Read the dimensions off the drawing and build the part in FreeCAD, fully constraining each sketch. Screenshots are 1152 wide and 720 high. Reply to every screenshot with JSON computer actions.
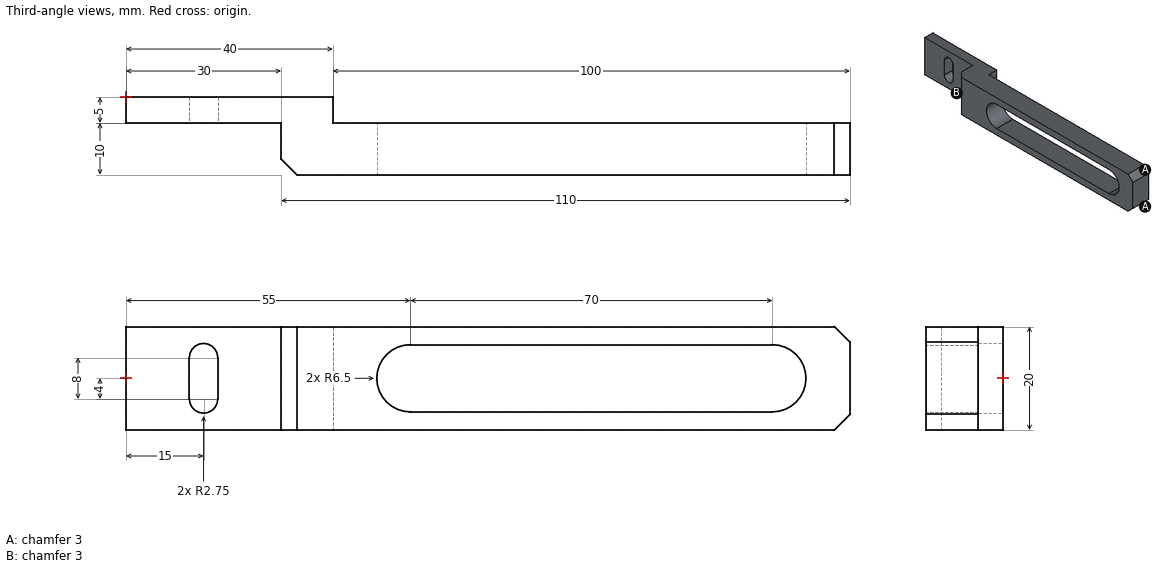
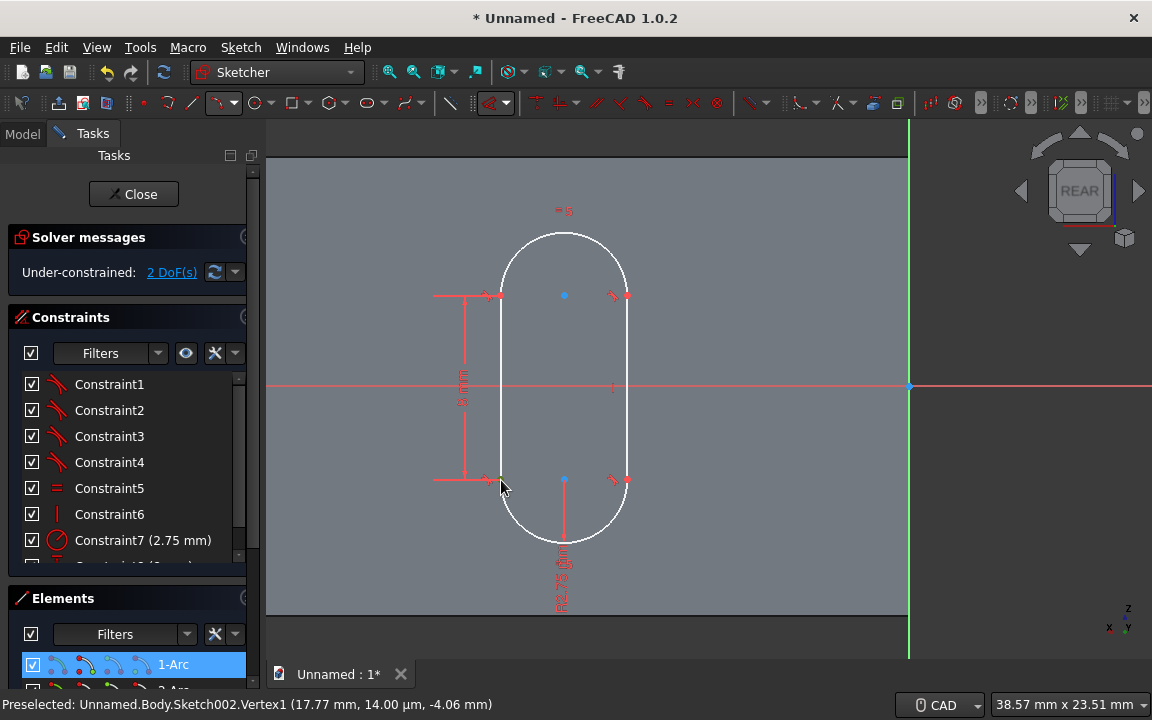
{"action": "key", "text": "i"}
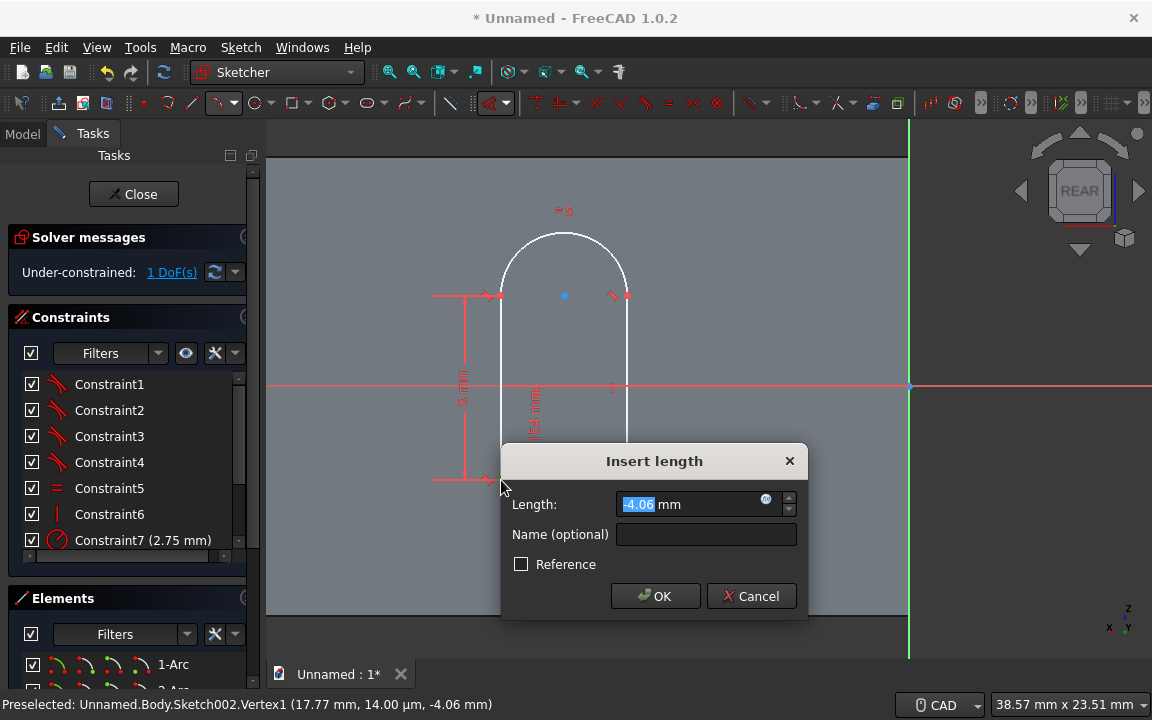
{"action": "type", "text": "-4"}
{"action": "key", "text": "Return"}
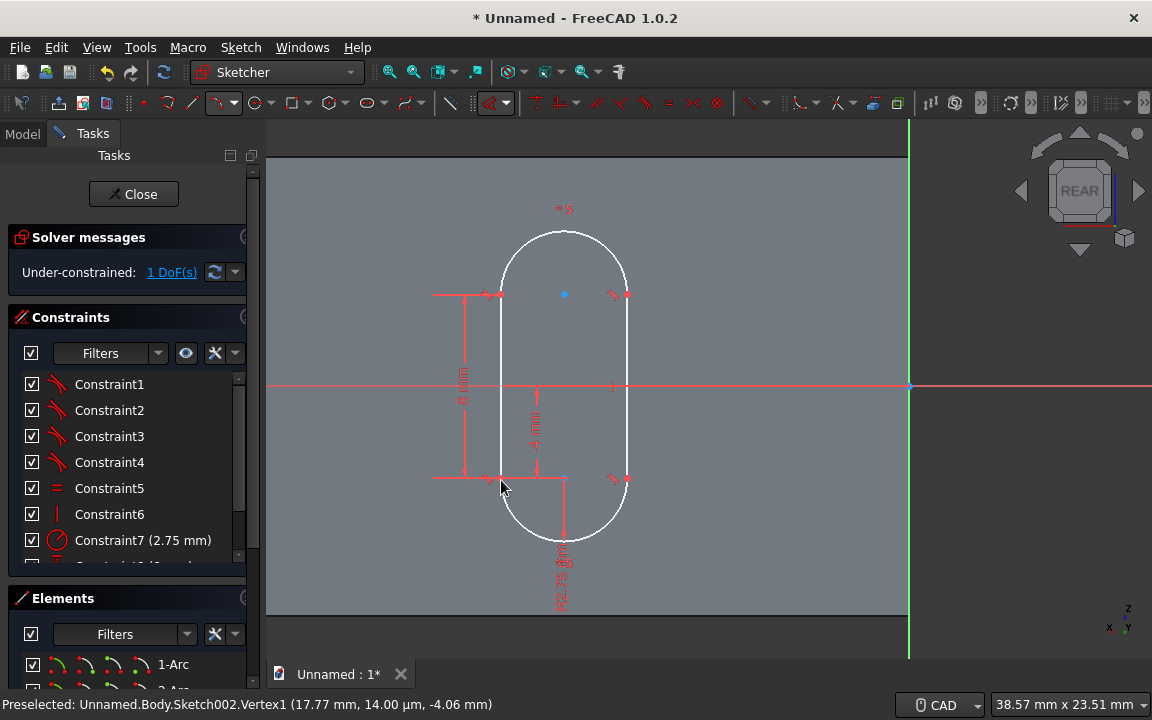
{"action": "left_click", "coordinate": [564, 478]}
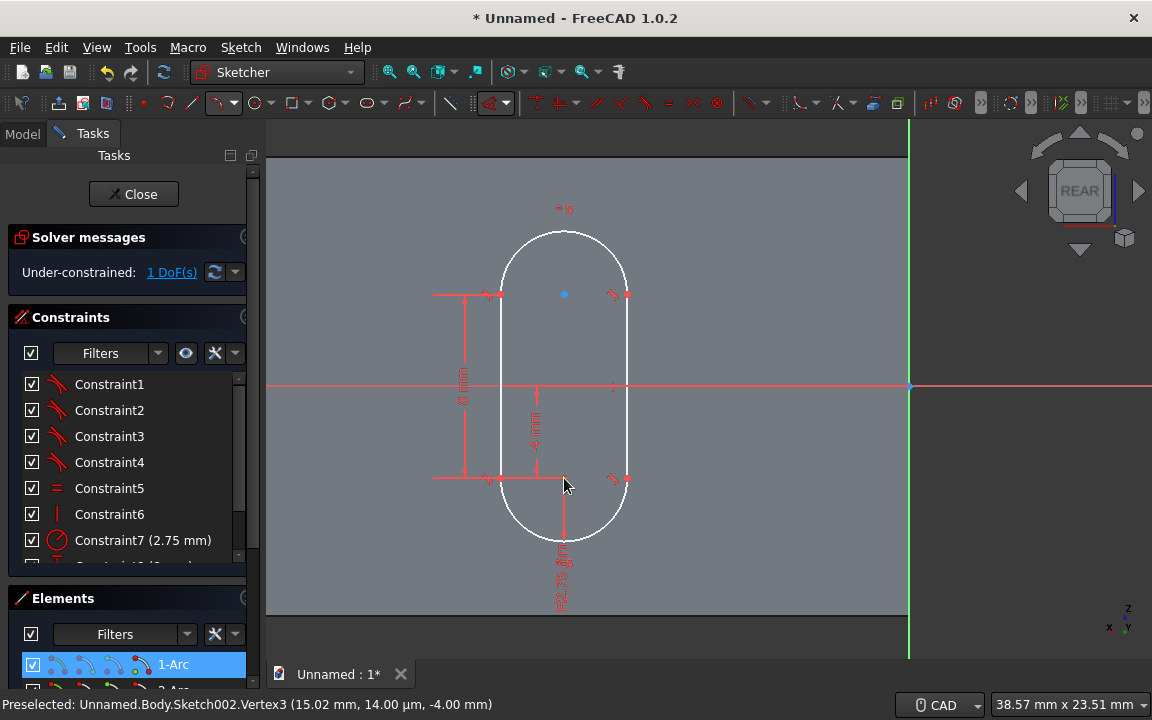
{"action": "key", "text": "l"}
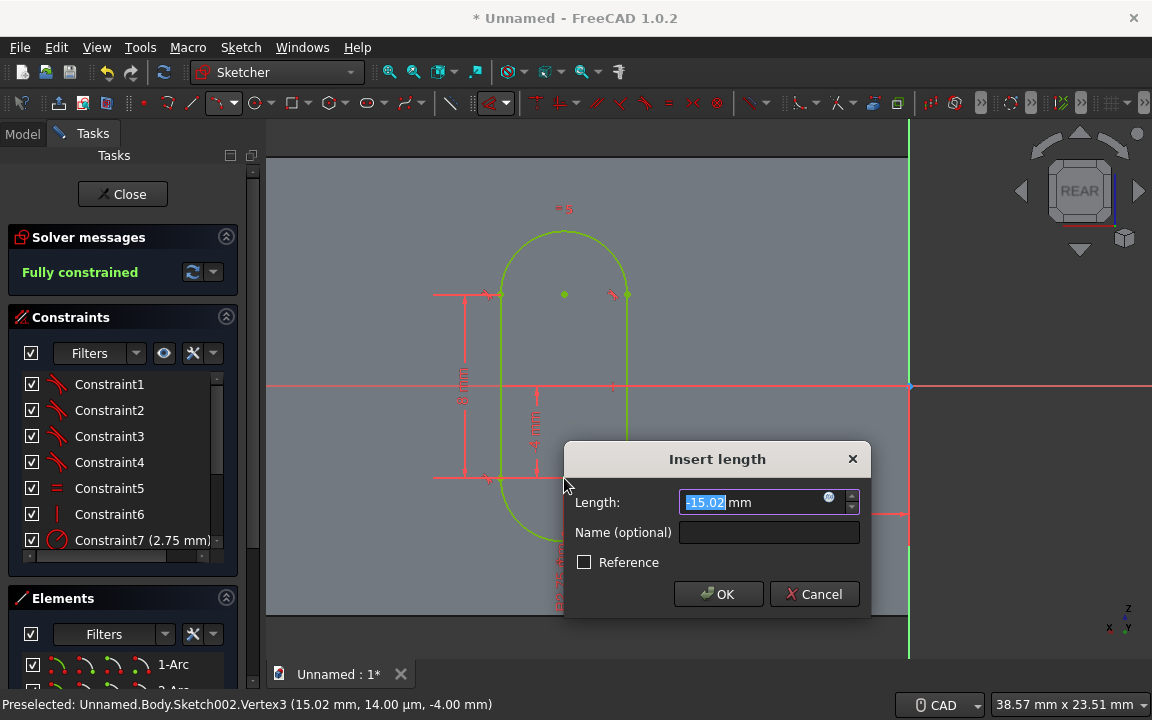
{"action": "type", "text": "-15"}
{"action": "key", "text": "Return"}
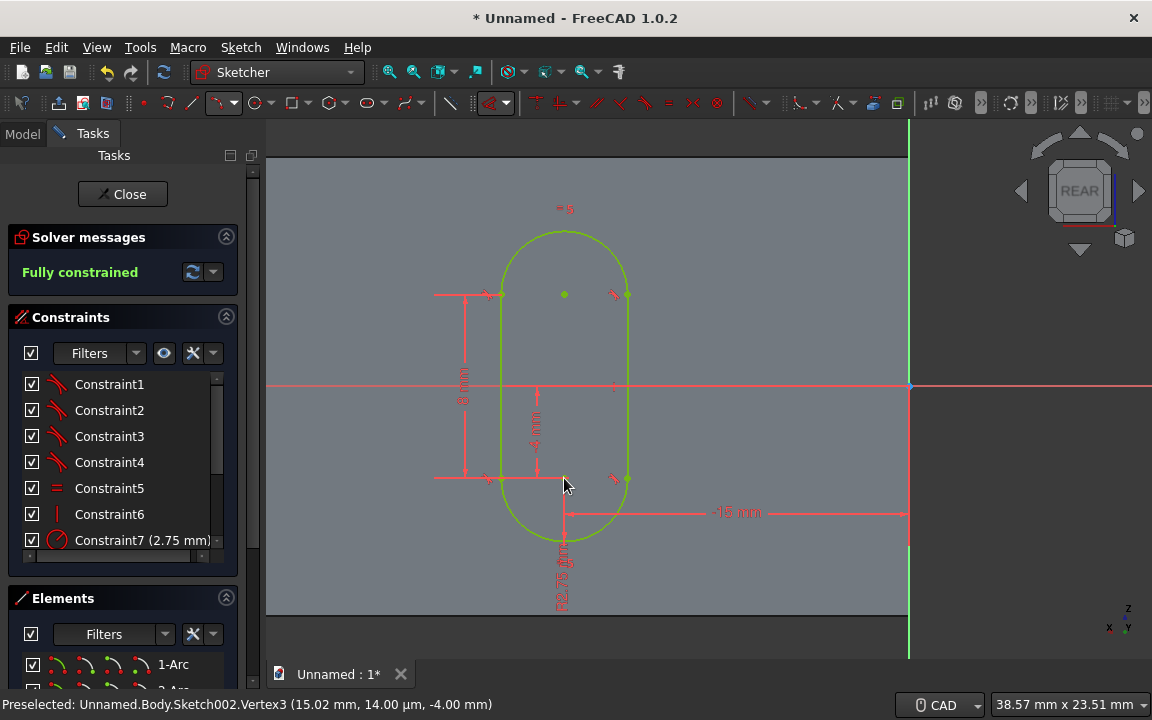
{"action": "left_click", "coordinate": [123, 194]}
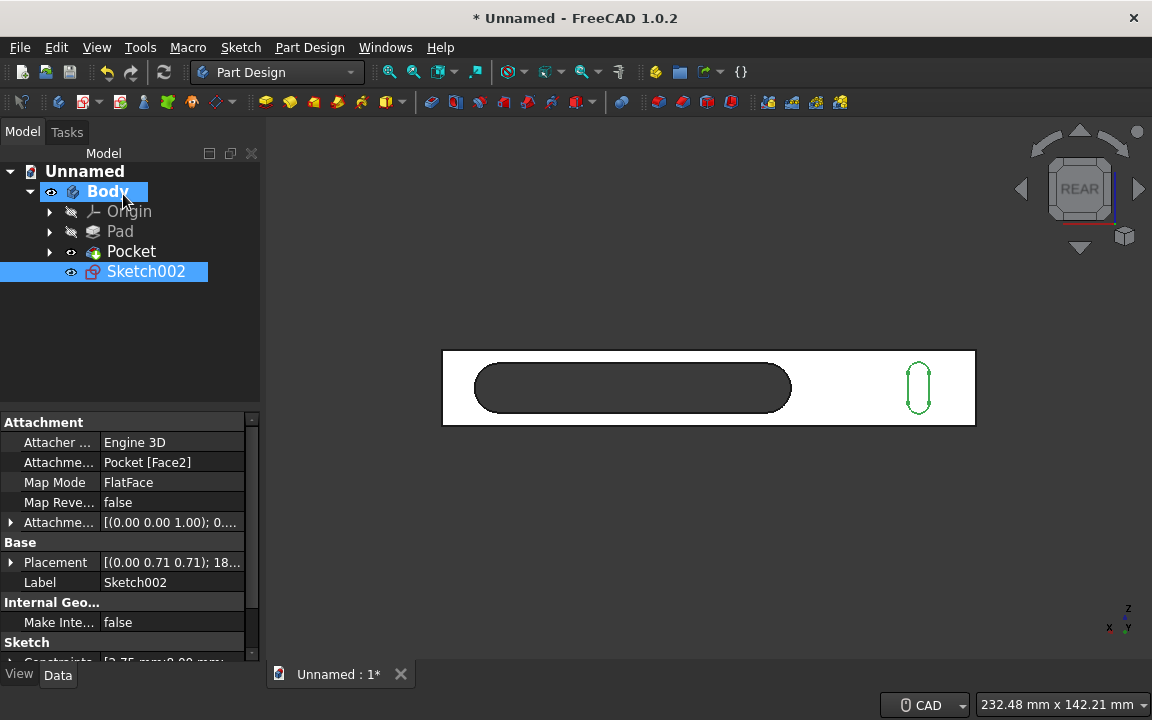
{"action": "left_click", "coordinate": [432, 102]}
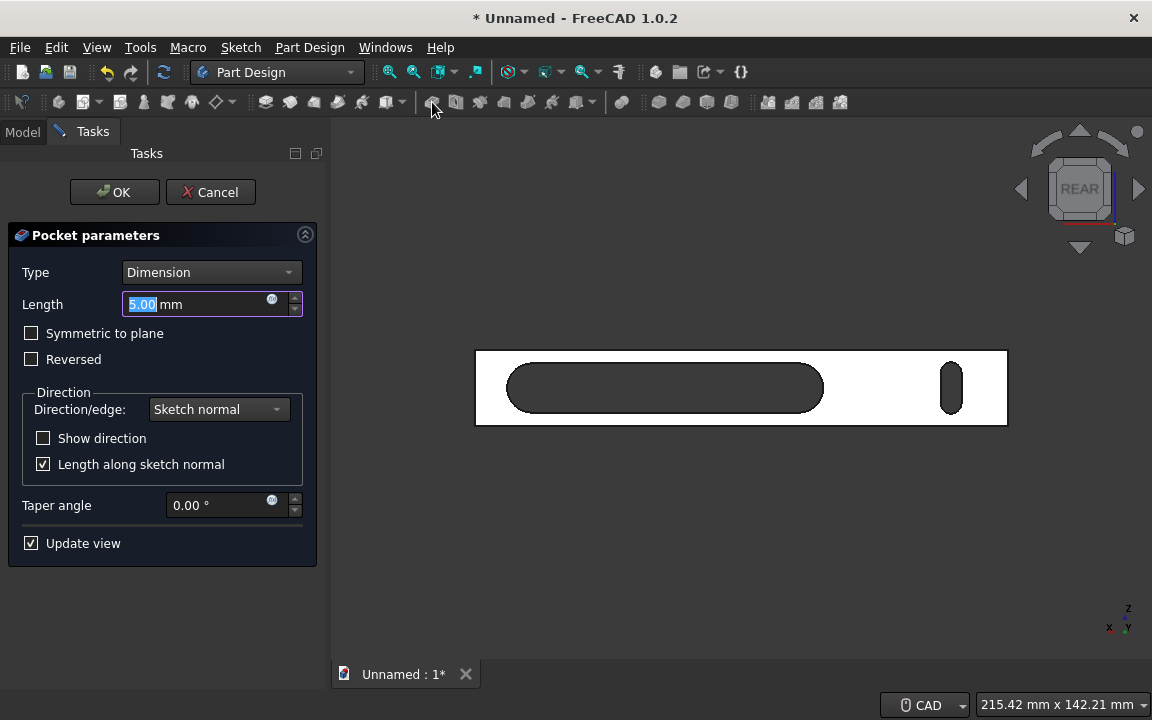
{"action": "left_click", "coordinate": [212, 272]}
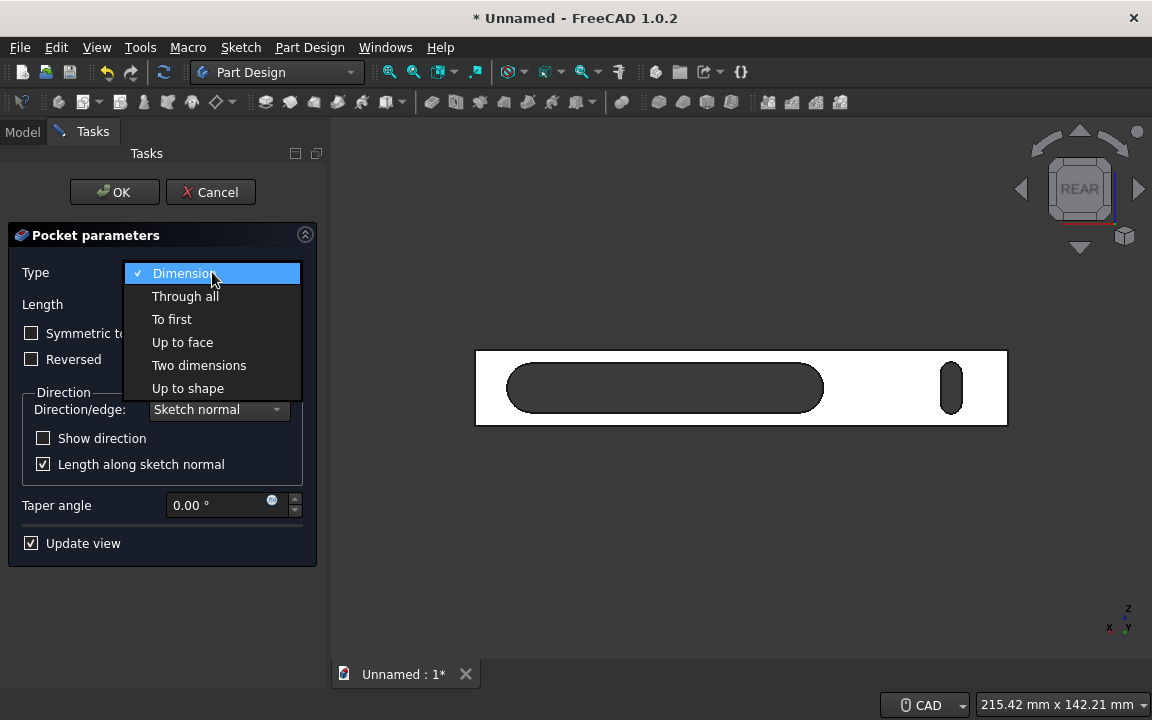
{"action": "left_click", "coordinate": [212, 296]}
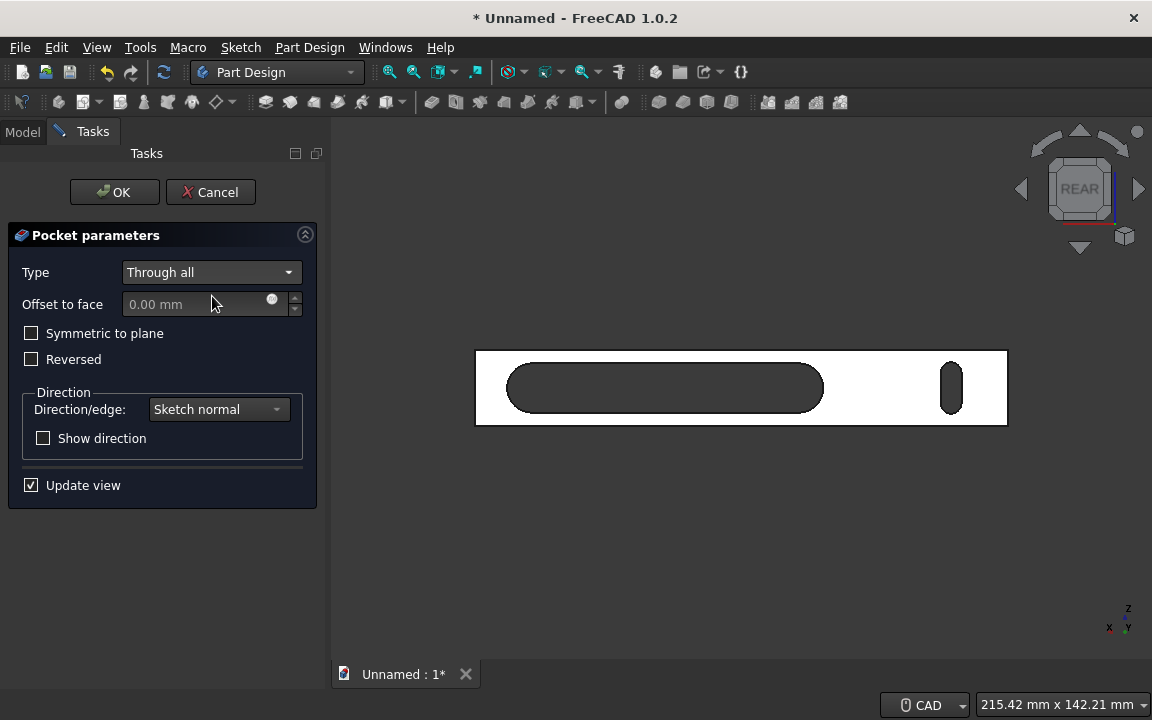
{"action": "left_click", "coordinate": [115, 192]}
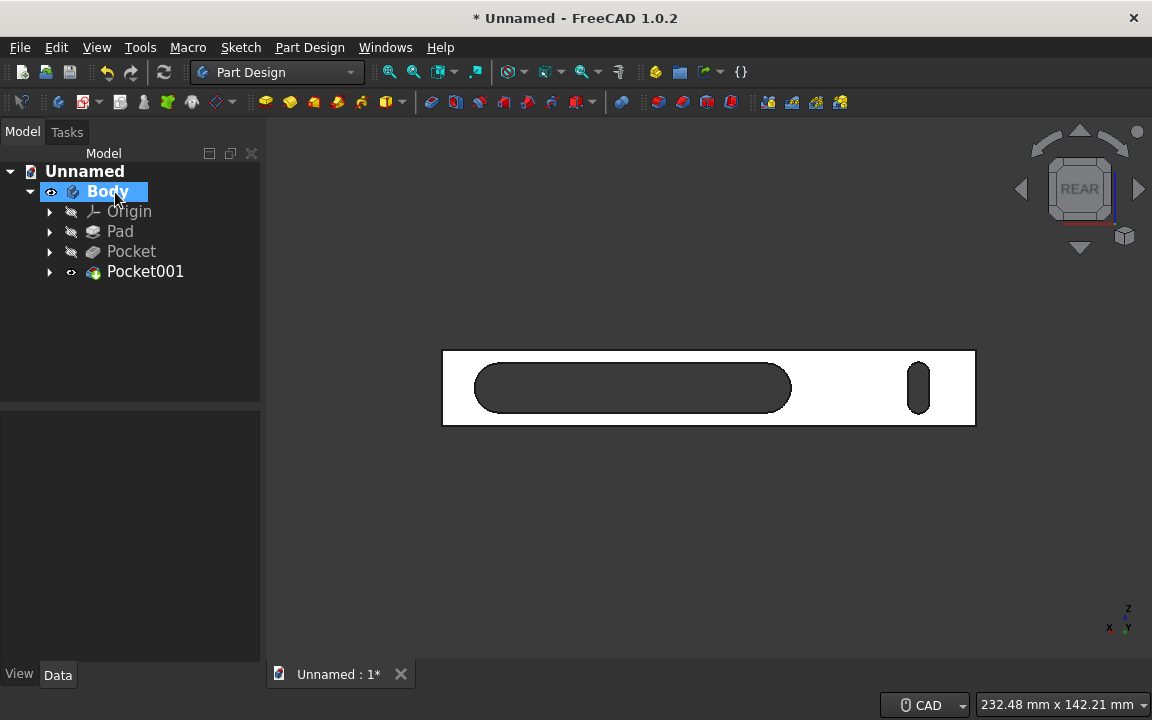
{"action": "key", "text": "0"}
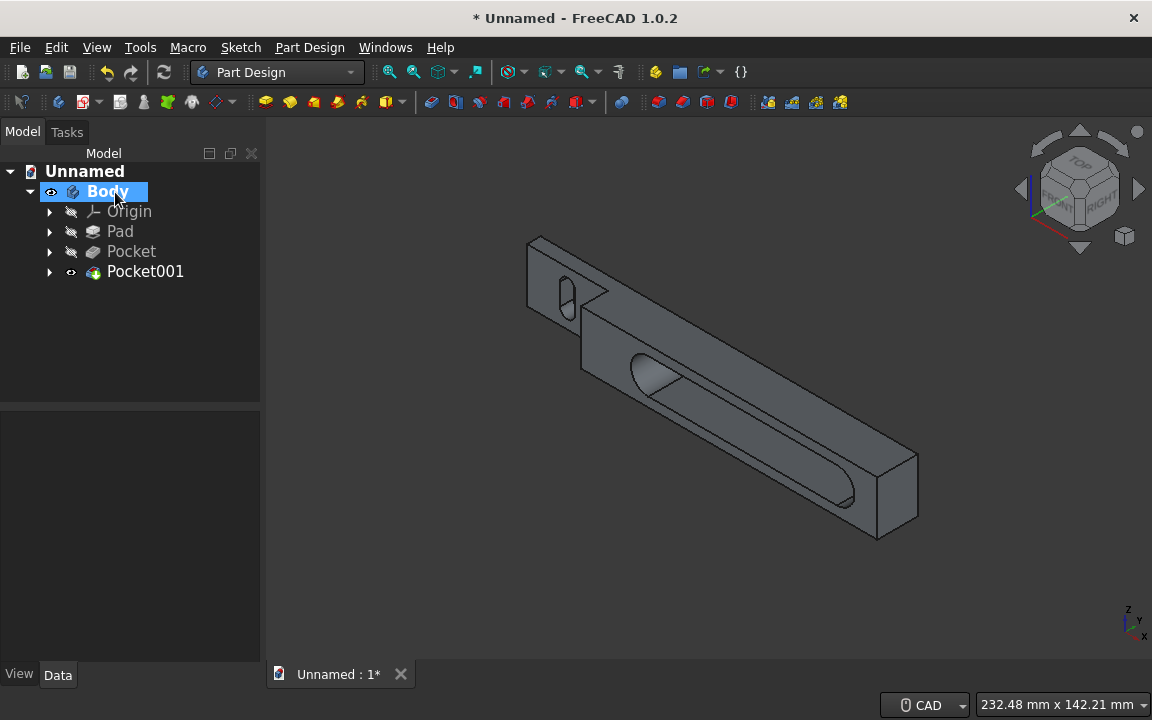
{"action": "left_click", "coordinate": [898, 465]}